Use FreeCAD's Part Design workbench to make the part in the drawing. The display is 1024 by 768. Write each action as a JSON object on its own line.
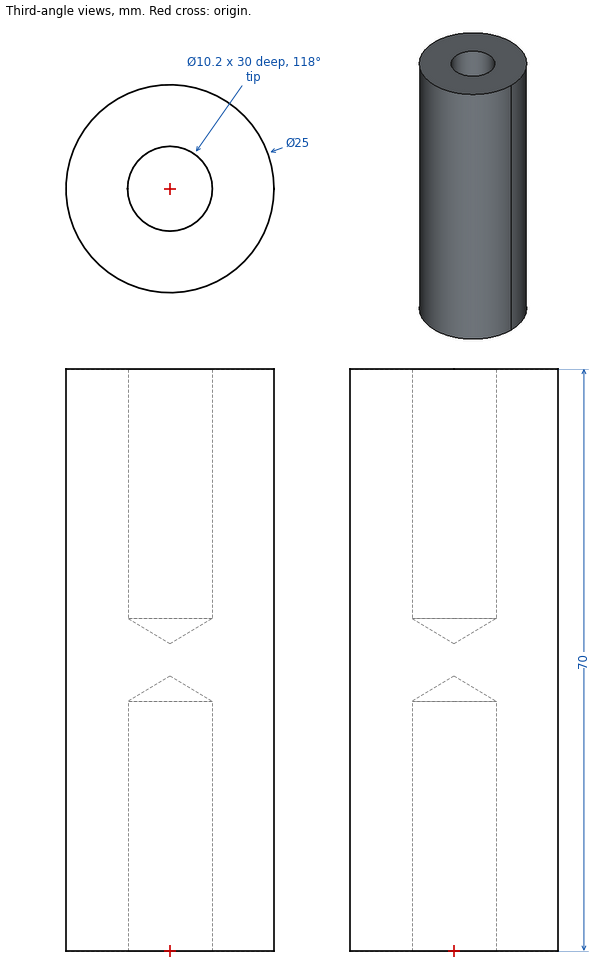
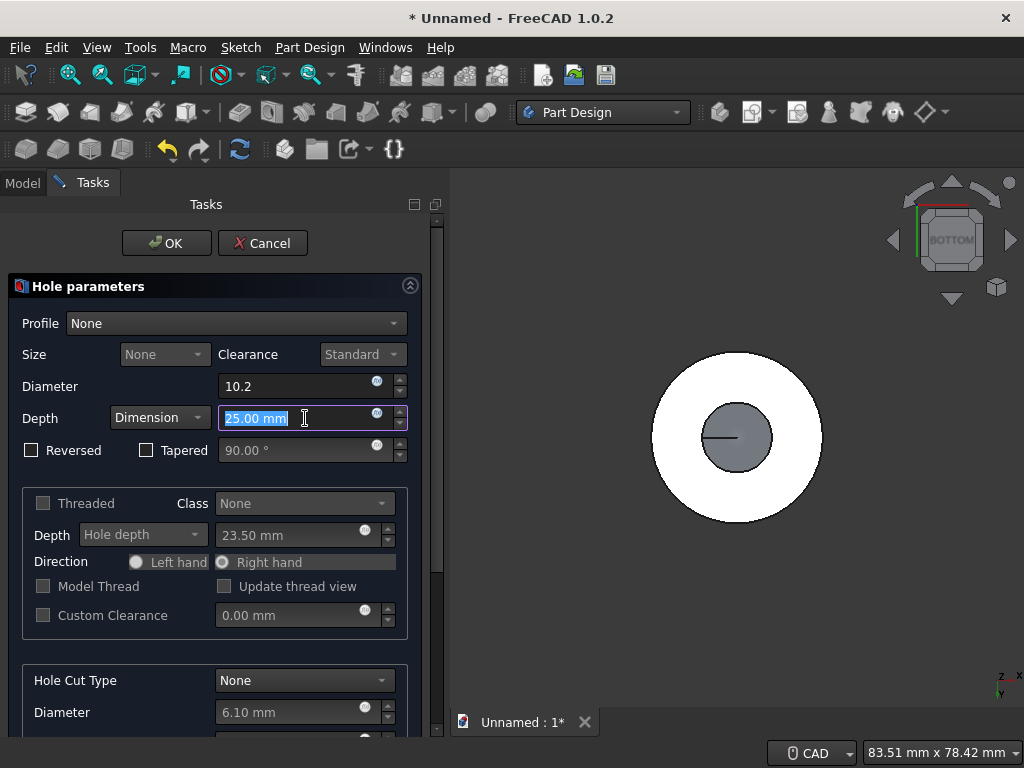
{"action": "type", "text": "30"}
{"action": "key", "text": "Tab"}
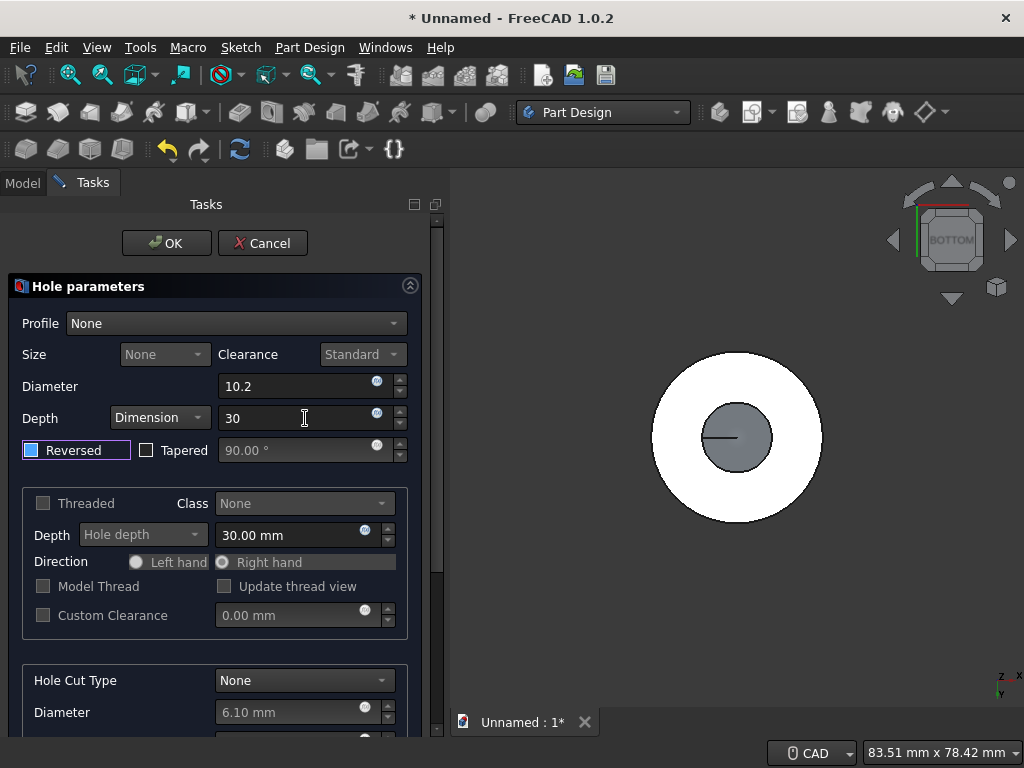
{"action": "left_click", "coordinate": [167, 243]}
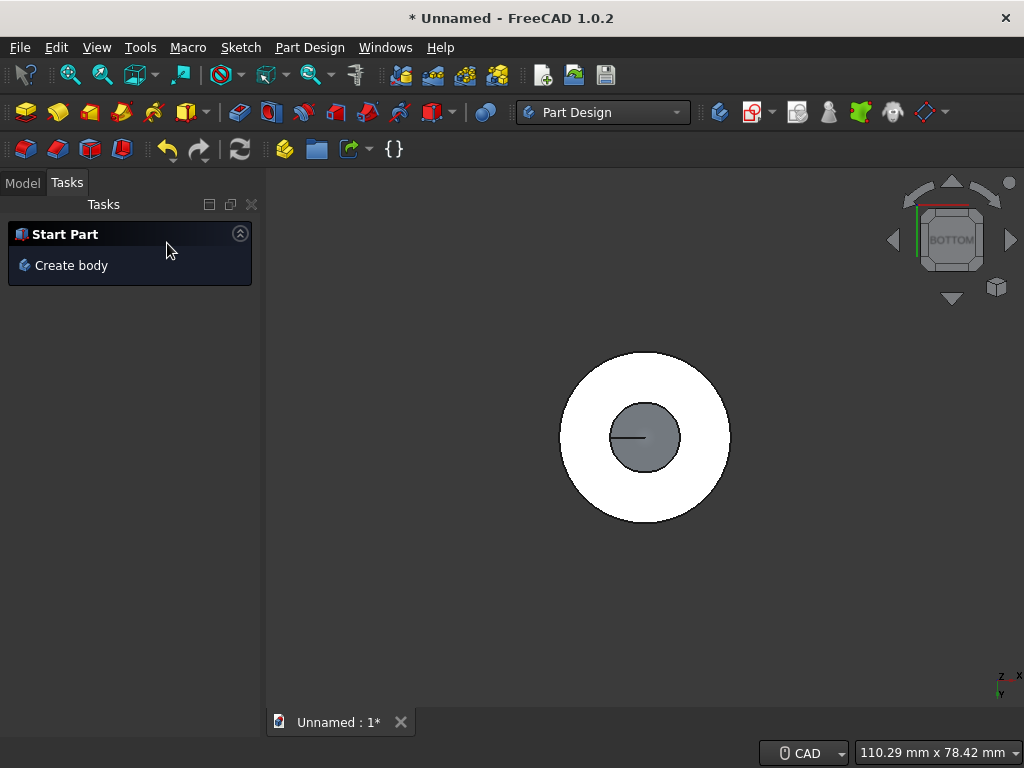
{"action": "key", "text": "0"}